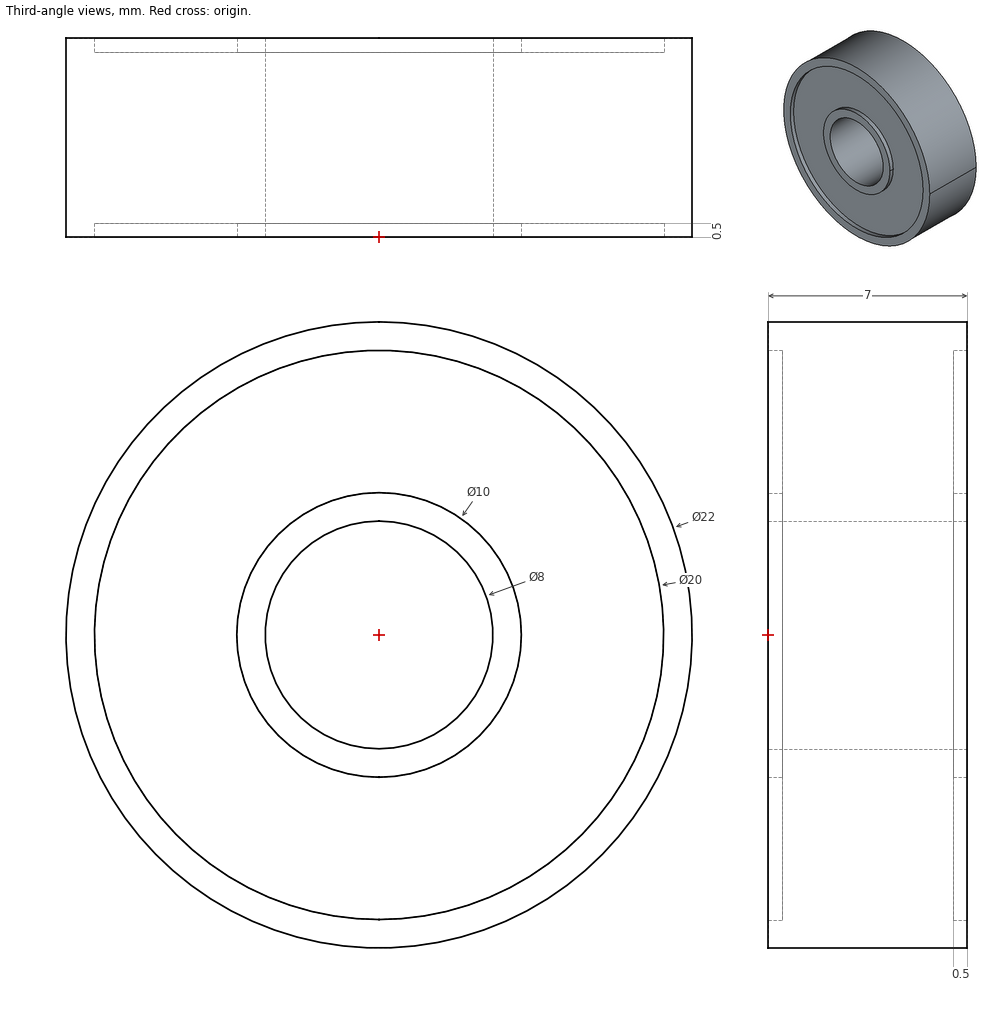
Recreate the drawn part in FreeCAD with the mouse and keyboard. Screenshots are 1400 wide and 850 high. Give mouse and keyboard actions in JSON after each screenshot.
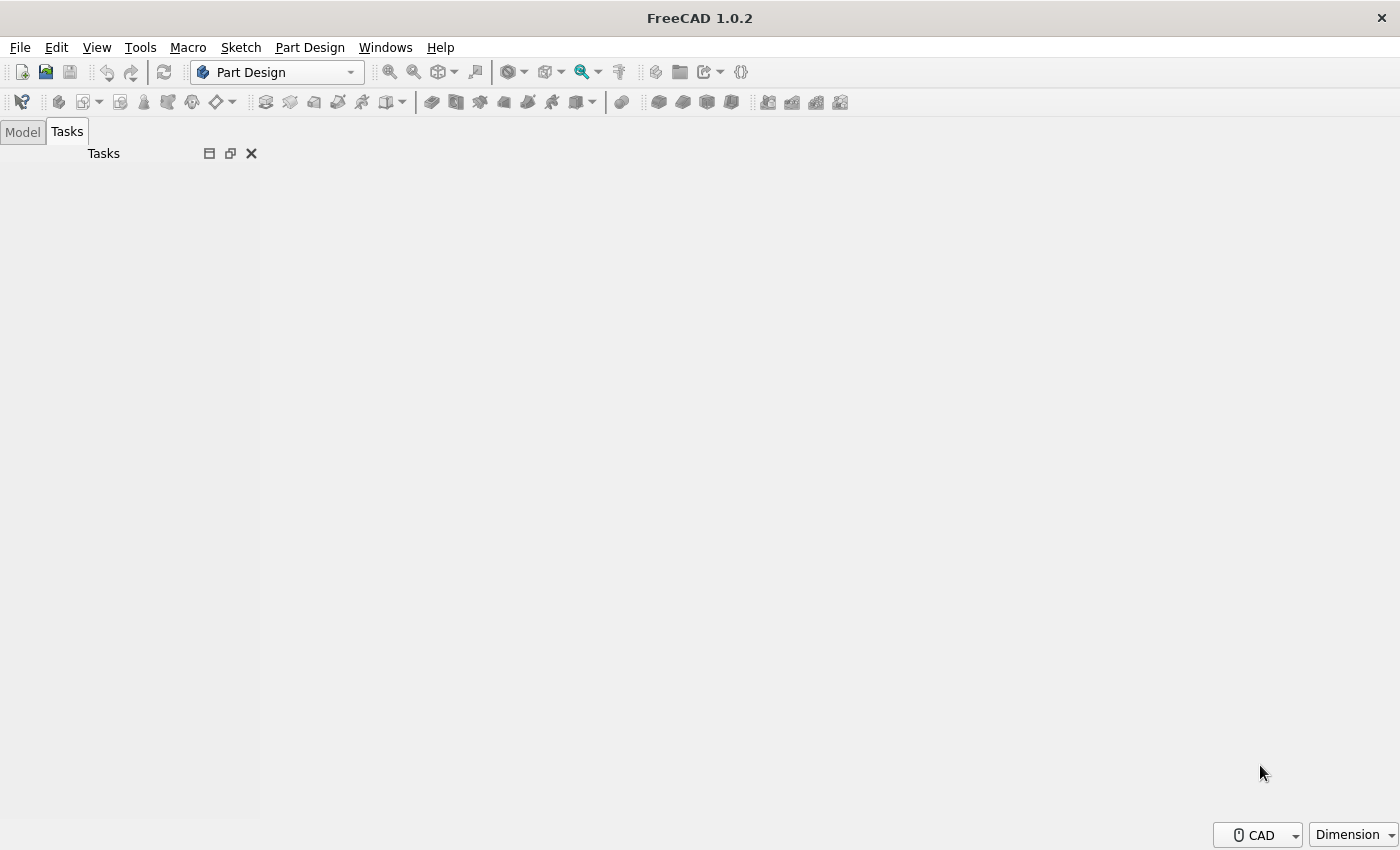
{"action": "key", "text": "ctrl+n"}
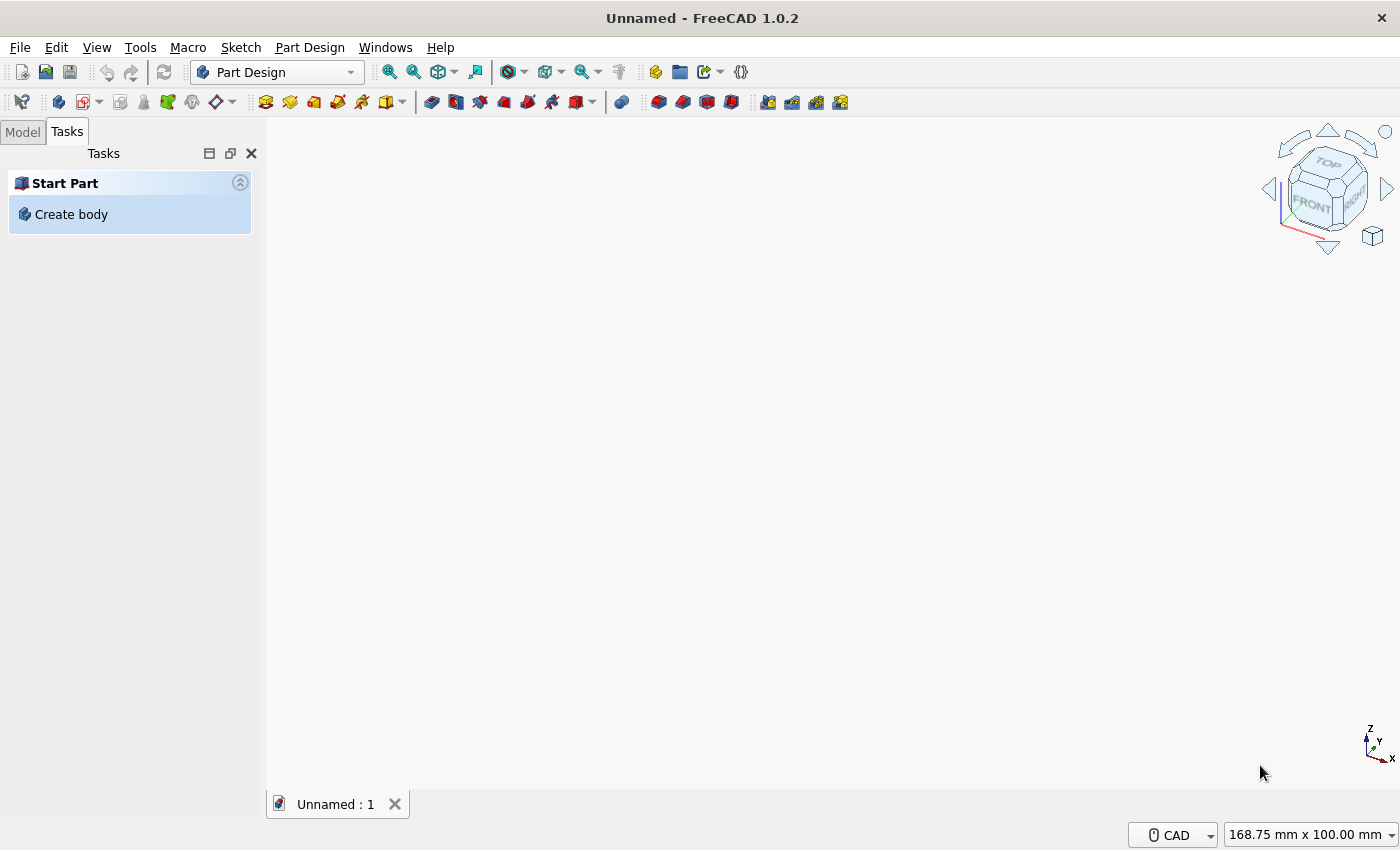
{"action": "left_click", "coordinate": [84, 102]}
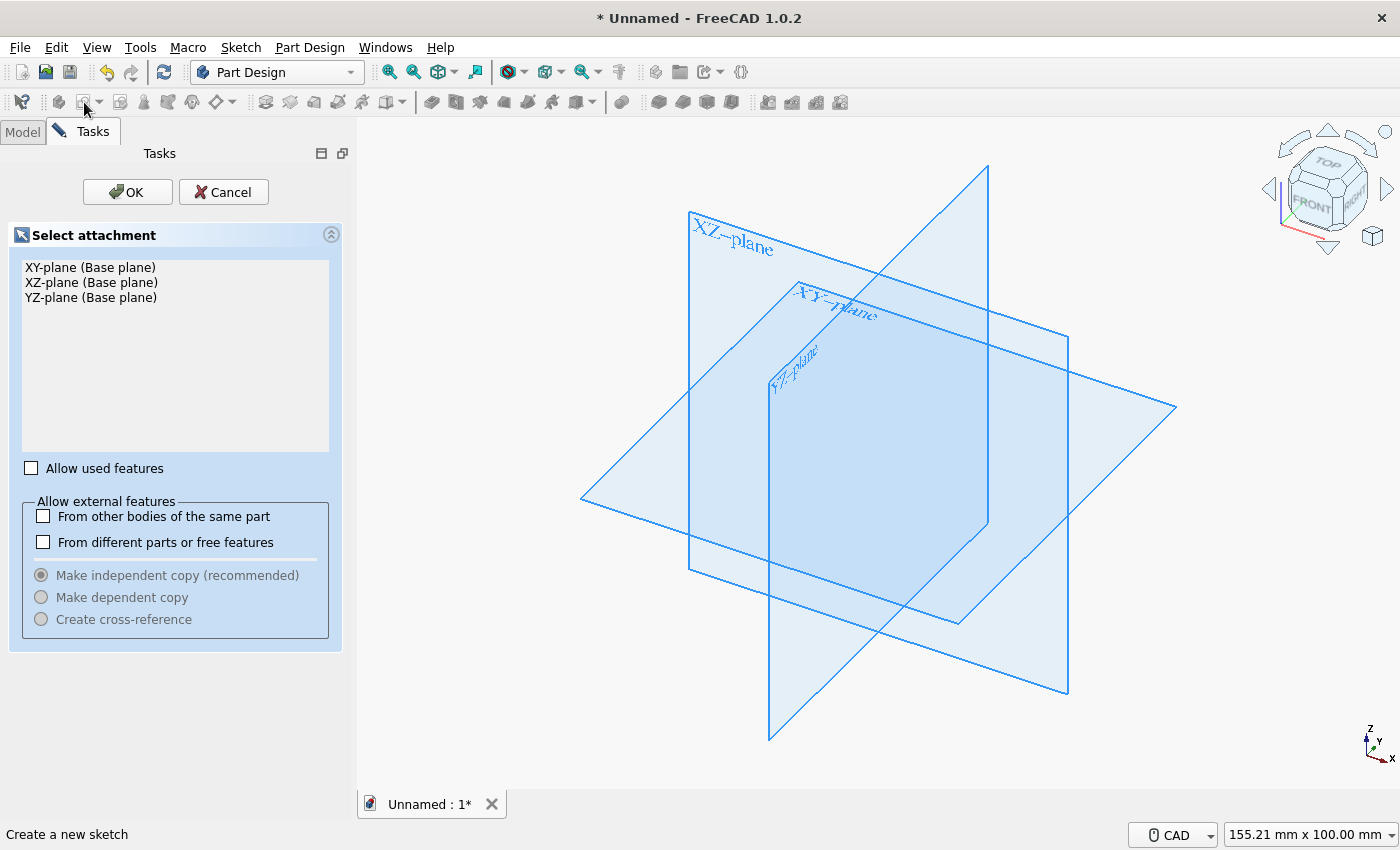
{"action": "left_click", "coordinate": [82, 282]}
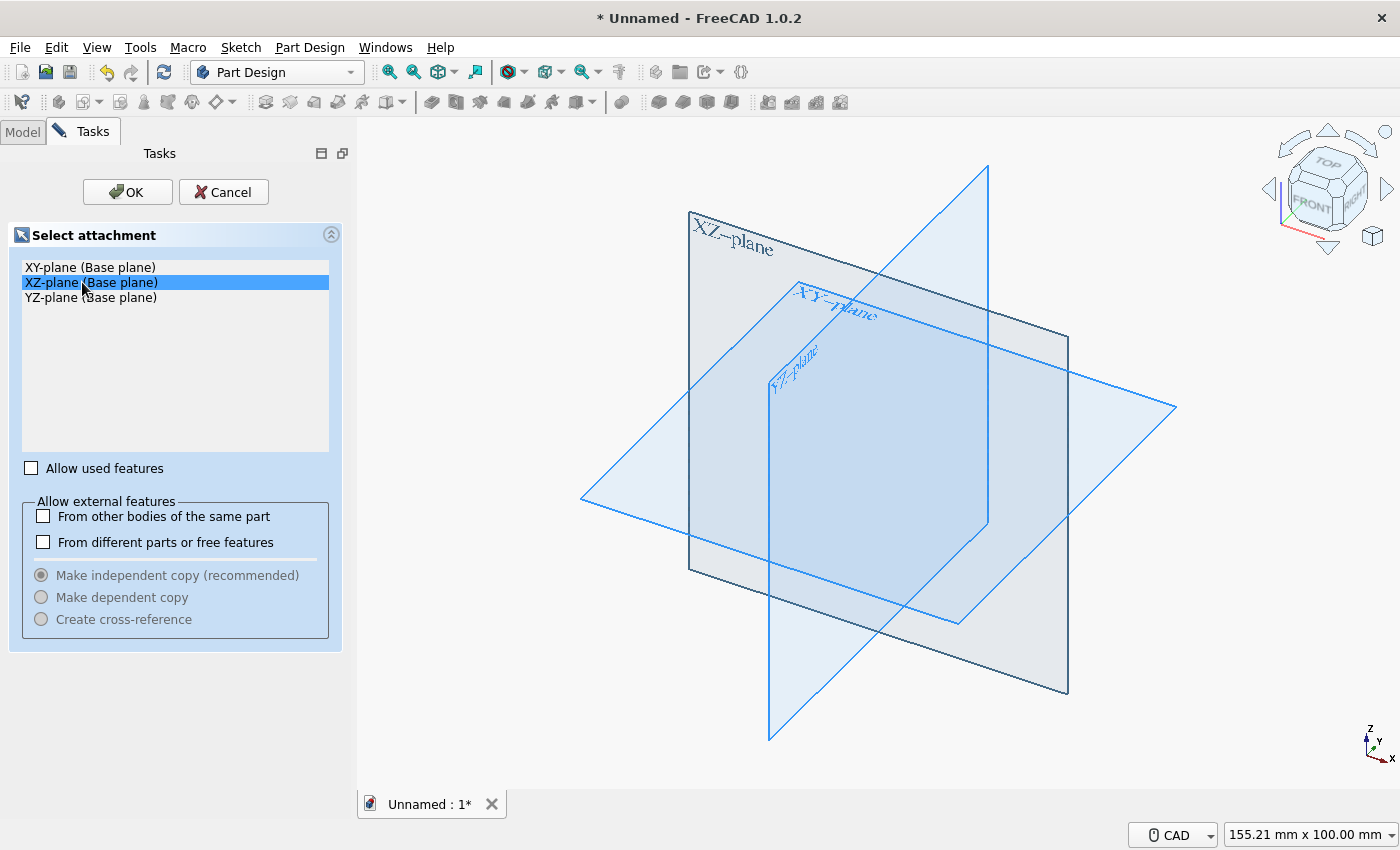
{"action": "left_click", "coordinate": [128, 192]}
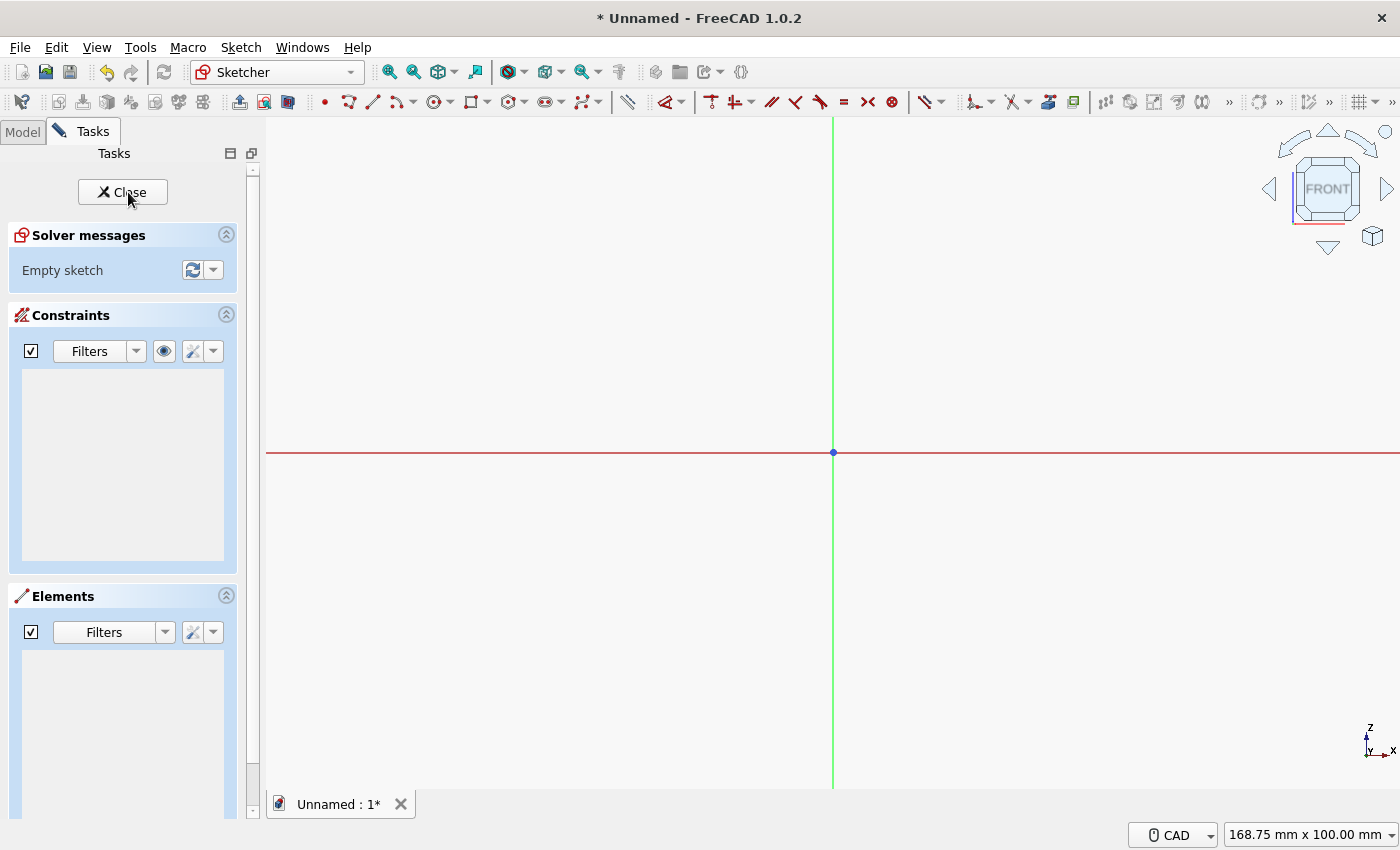
{"action": "scroll", "coordinate": [873, 453], "scroll_direction": "up", "scroll_amount": 5}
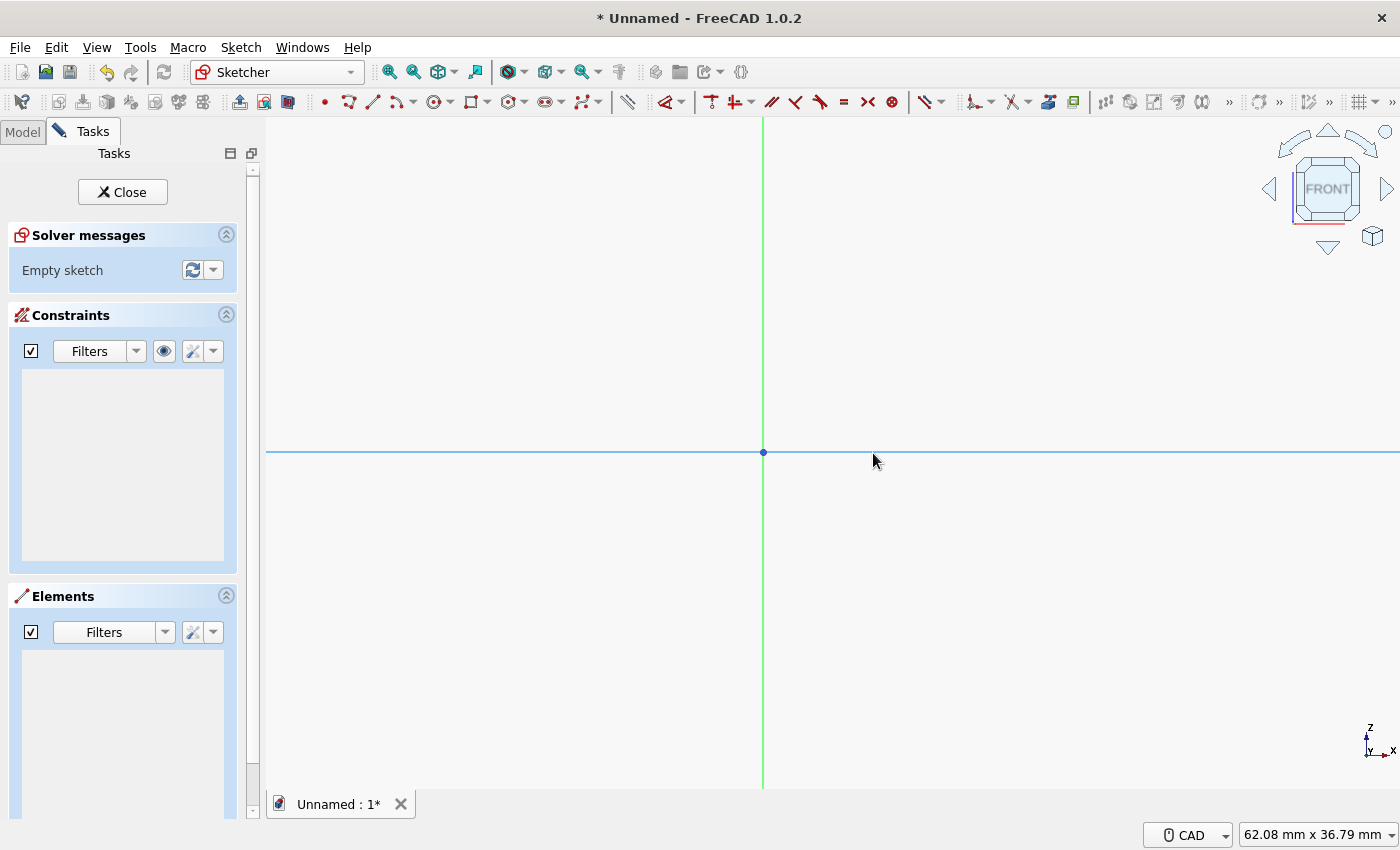
{"action": "key", "text": "g c"}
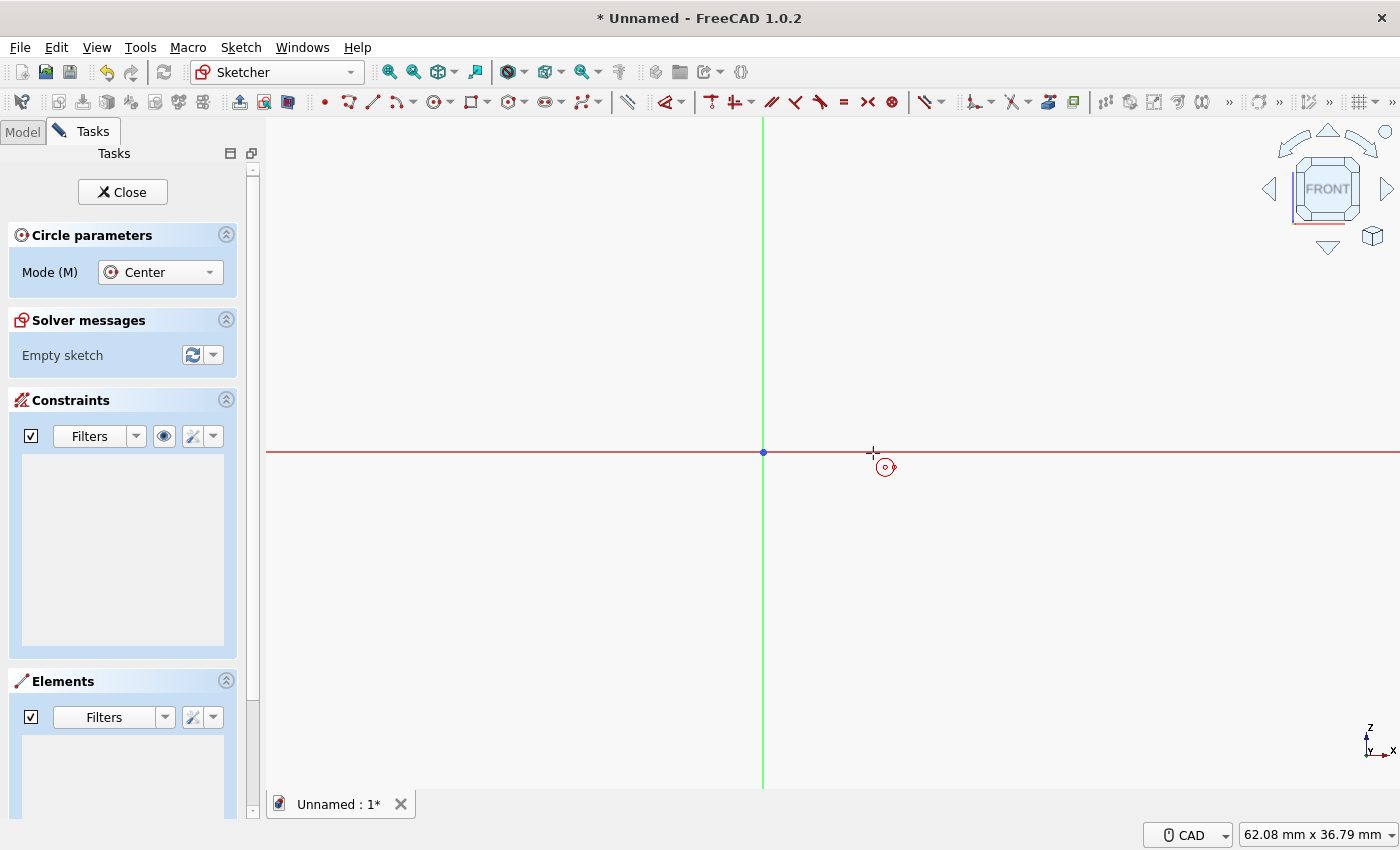
{"action": "left_click", "coordinate": [763, 452]}
{"action": "mouse_move", "coordinate": [905, 310]}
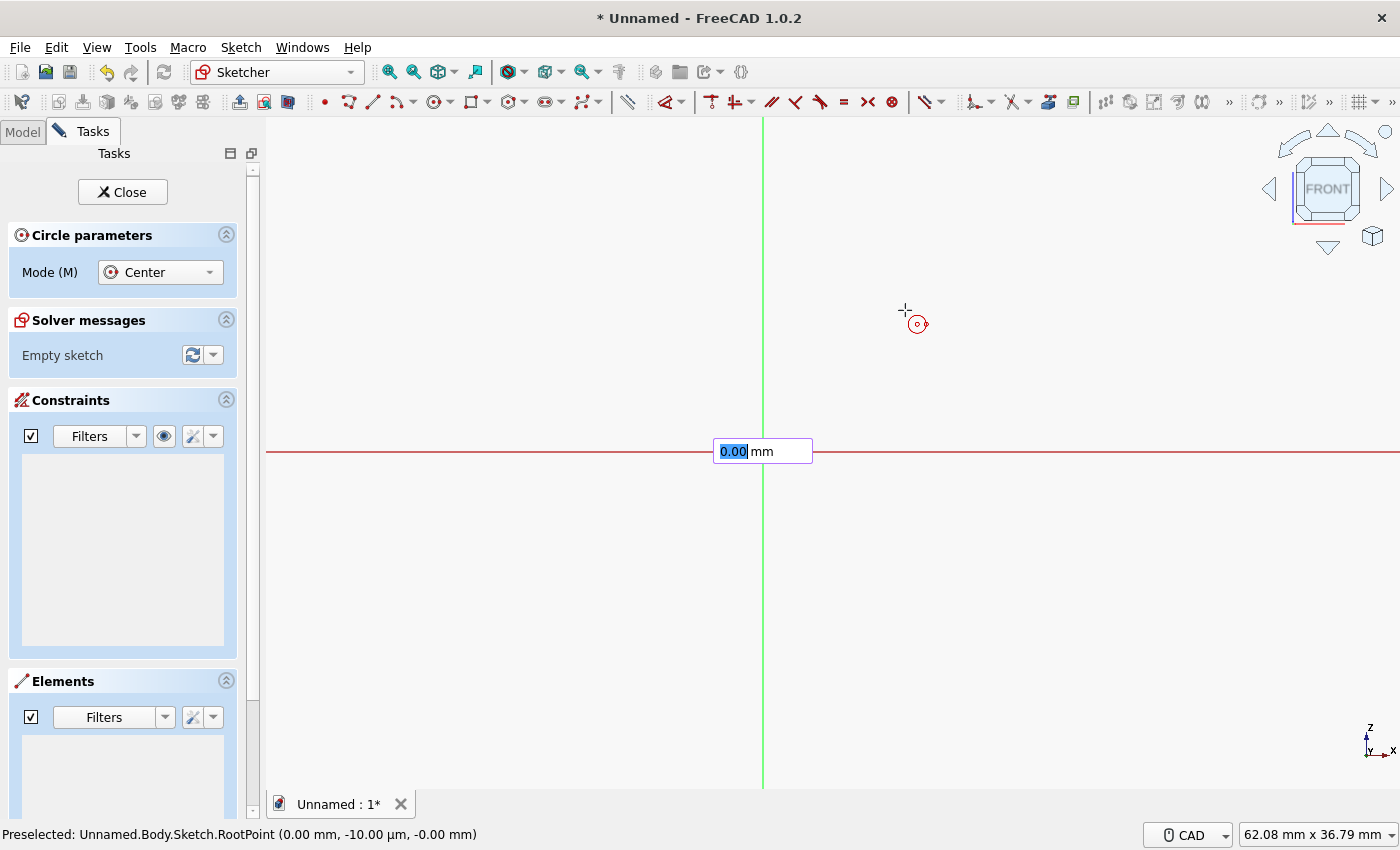
{"action": "type", "text": "22"}
{"action": "key", "text": "Return"}